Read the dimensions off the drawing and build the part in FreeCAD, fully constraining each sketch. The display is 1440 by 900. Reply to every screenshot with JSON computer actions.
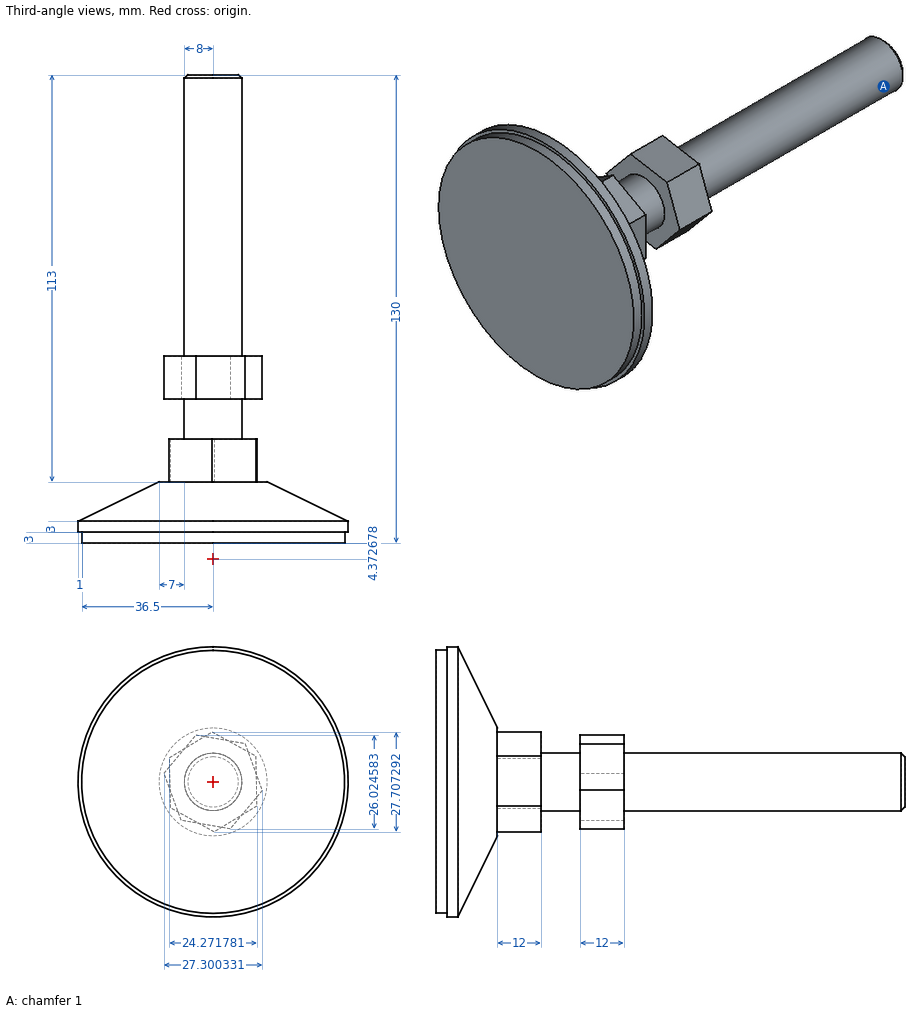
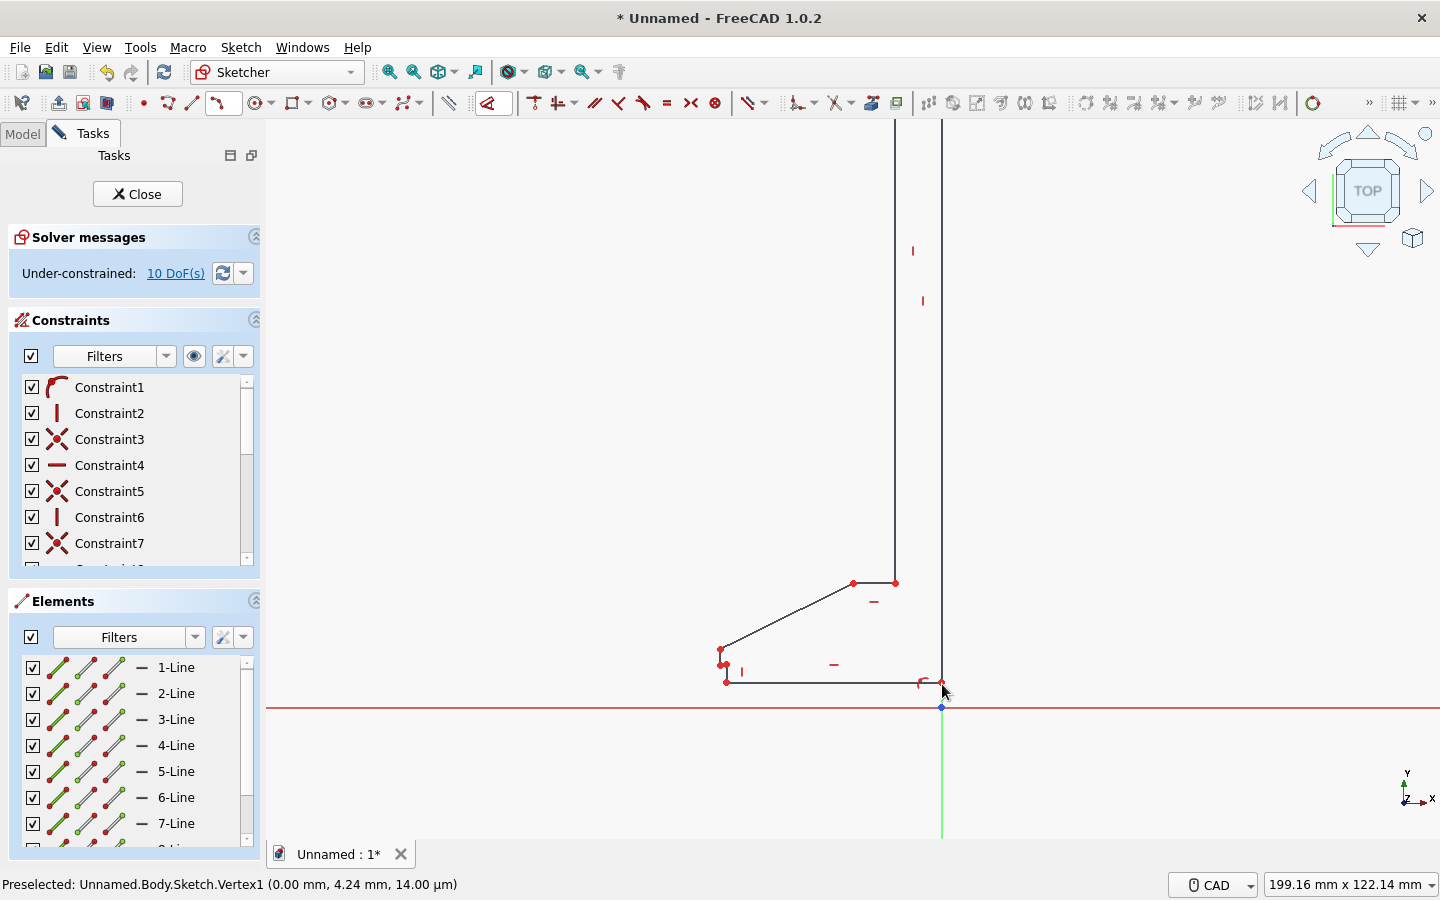
{"action": "scroll", "coordinate": [723, 665], "scroll_direction": "up", "scroll_amount": 8}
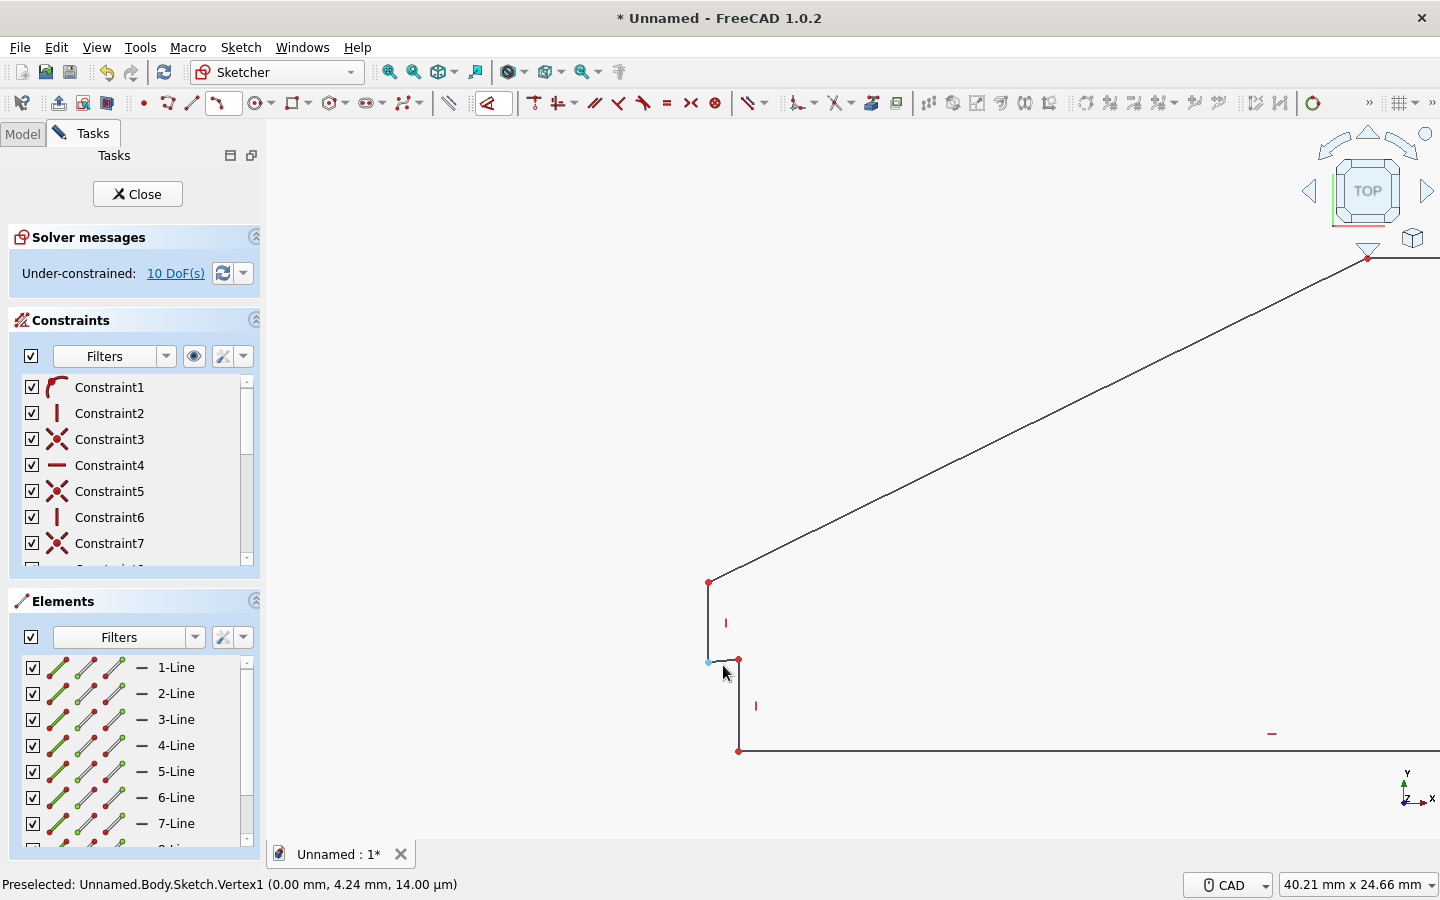
{"action": "left_click", "coordinate": [724, 661]}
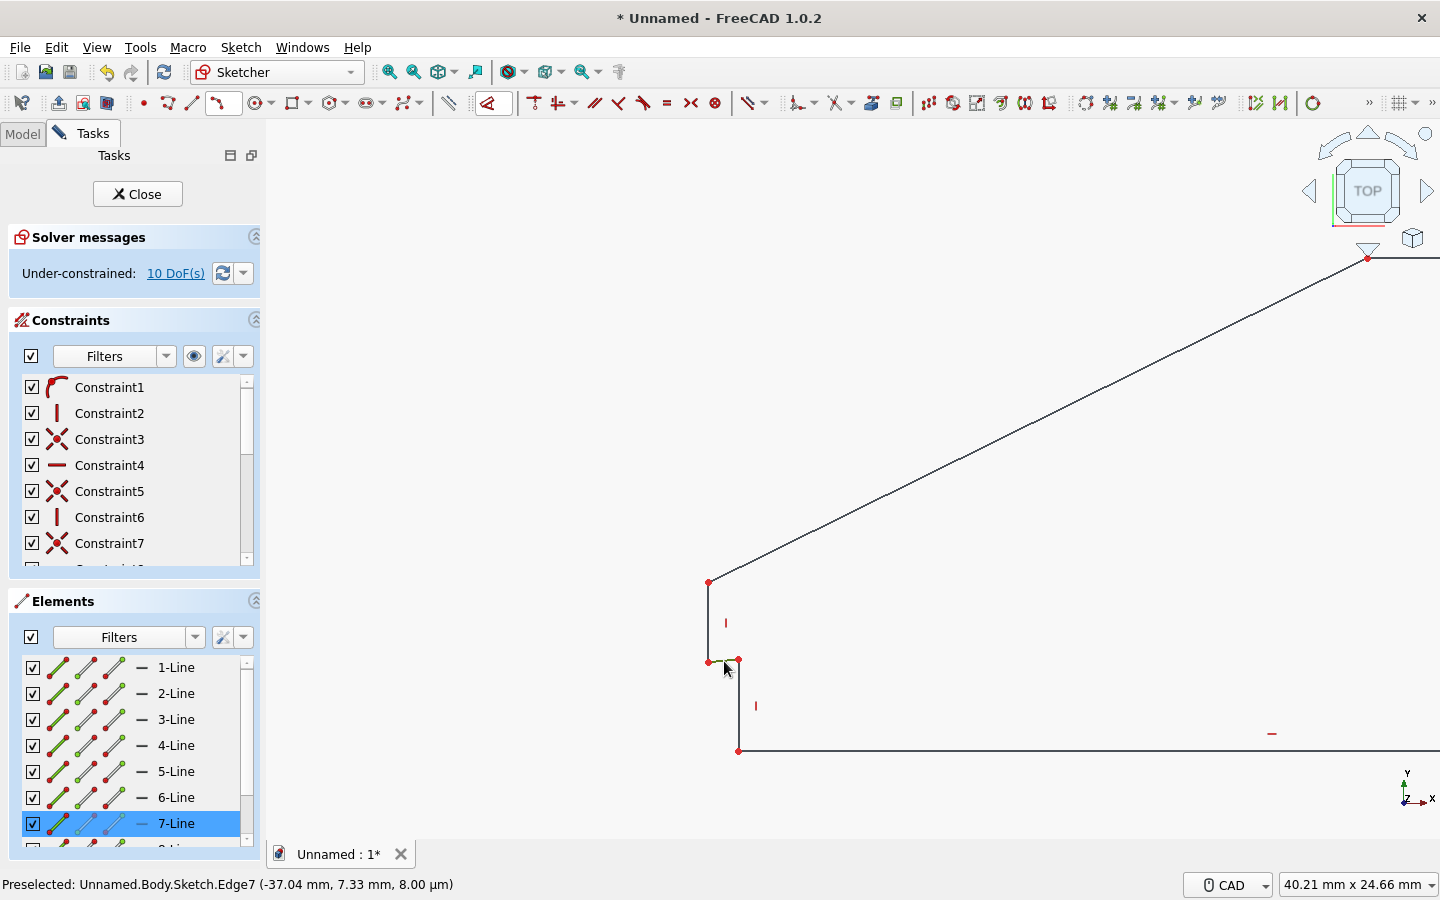
{"action": "key", "text": "h"}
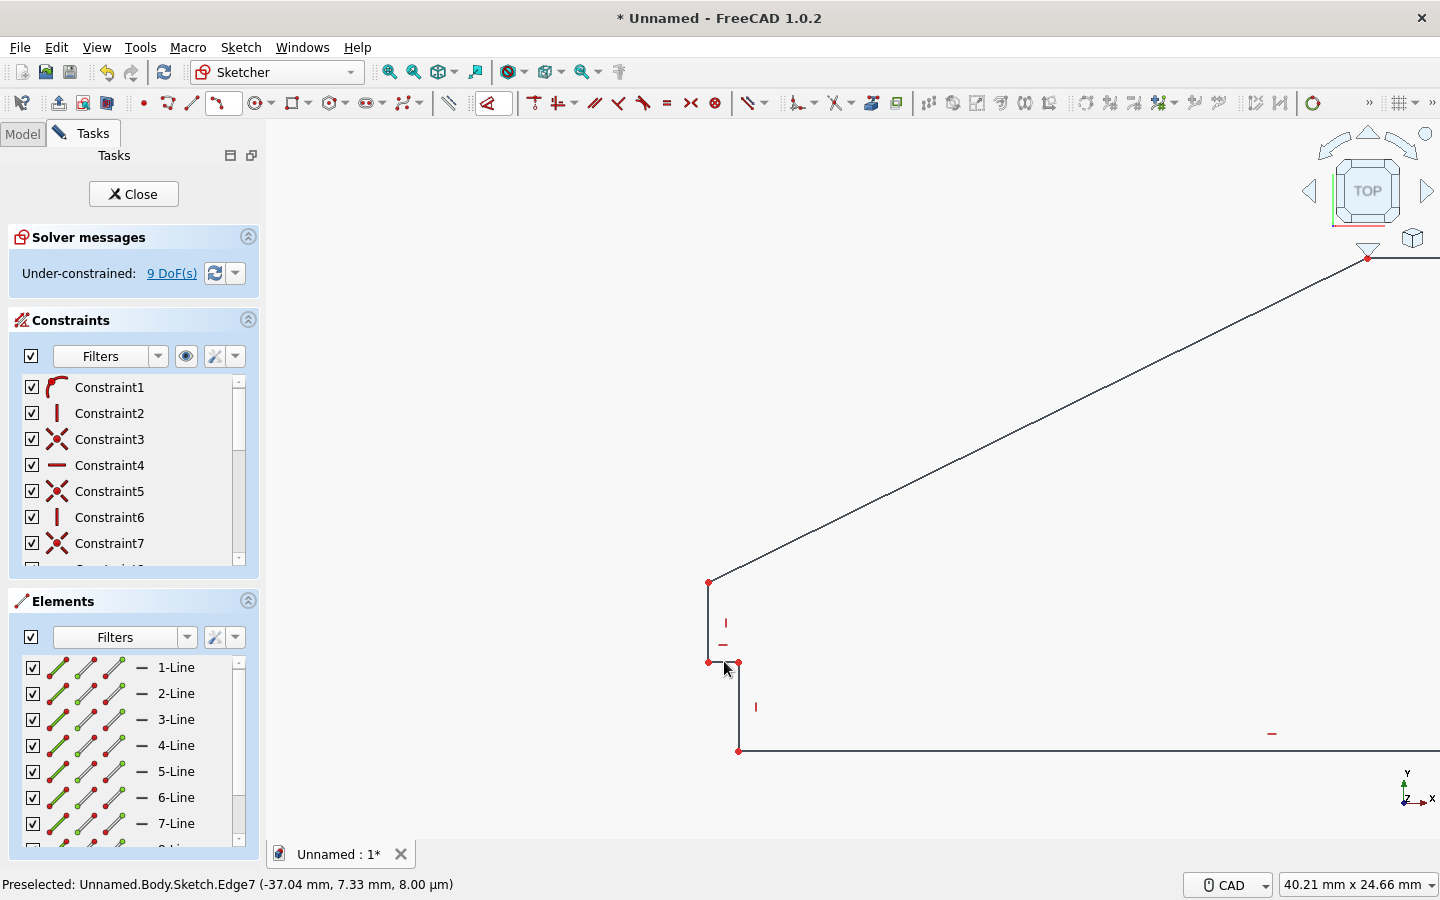
{"action": "scroll", "coordinate": [726, 674], "scroll_direction": "down", "scroll_amount": 11}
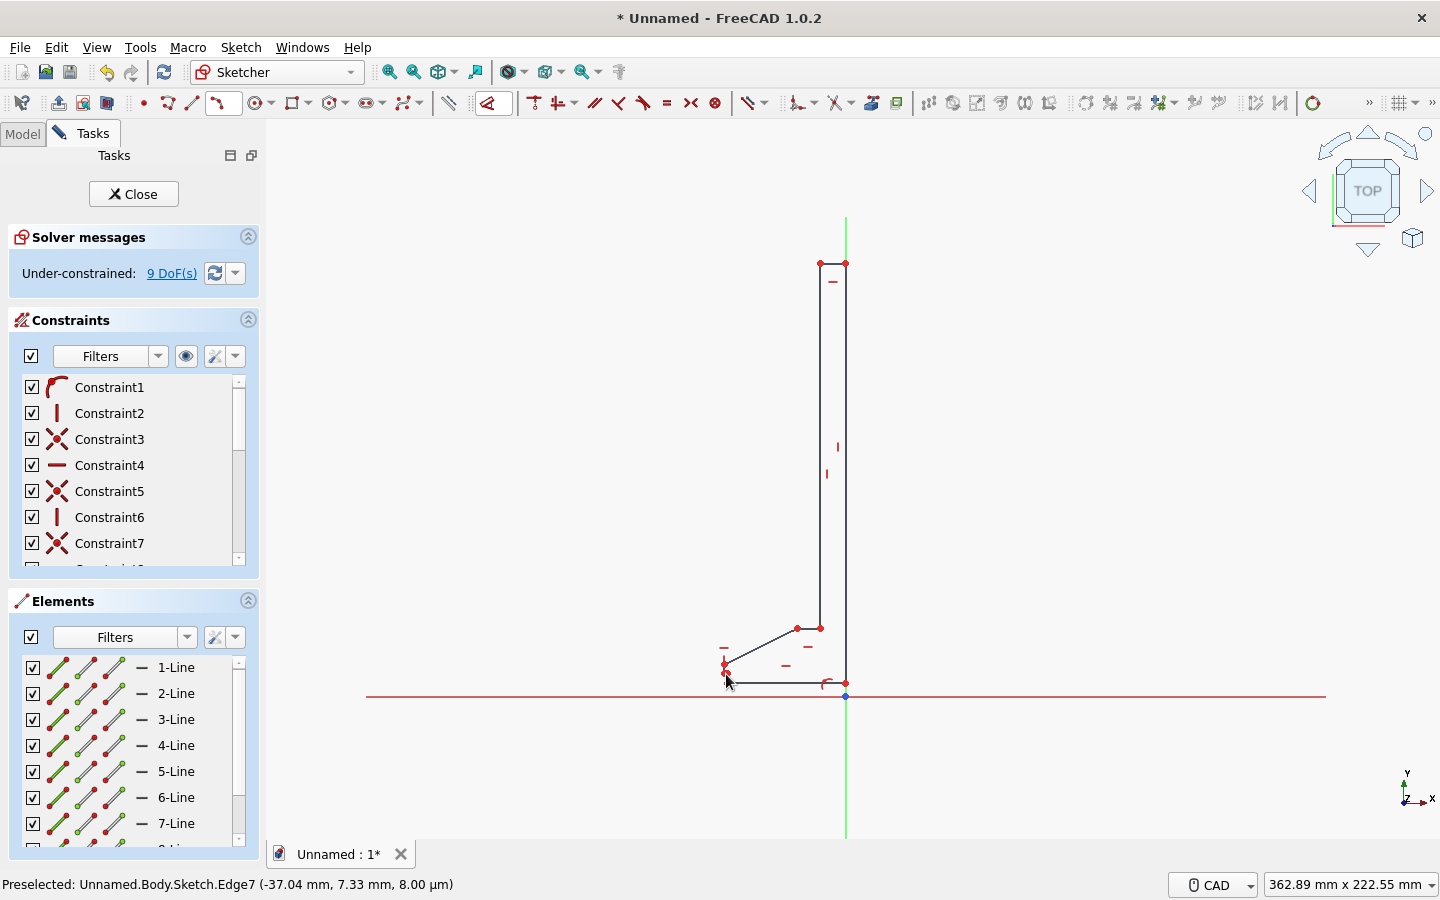
{"action": "scroll", "coordinate": [838, 264], "scroll_direction": "up", "scroll_amount": 3}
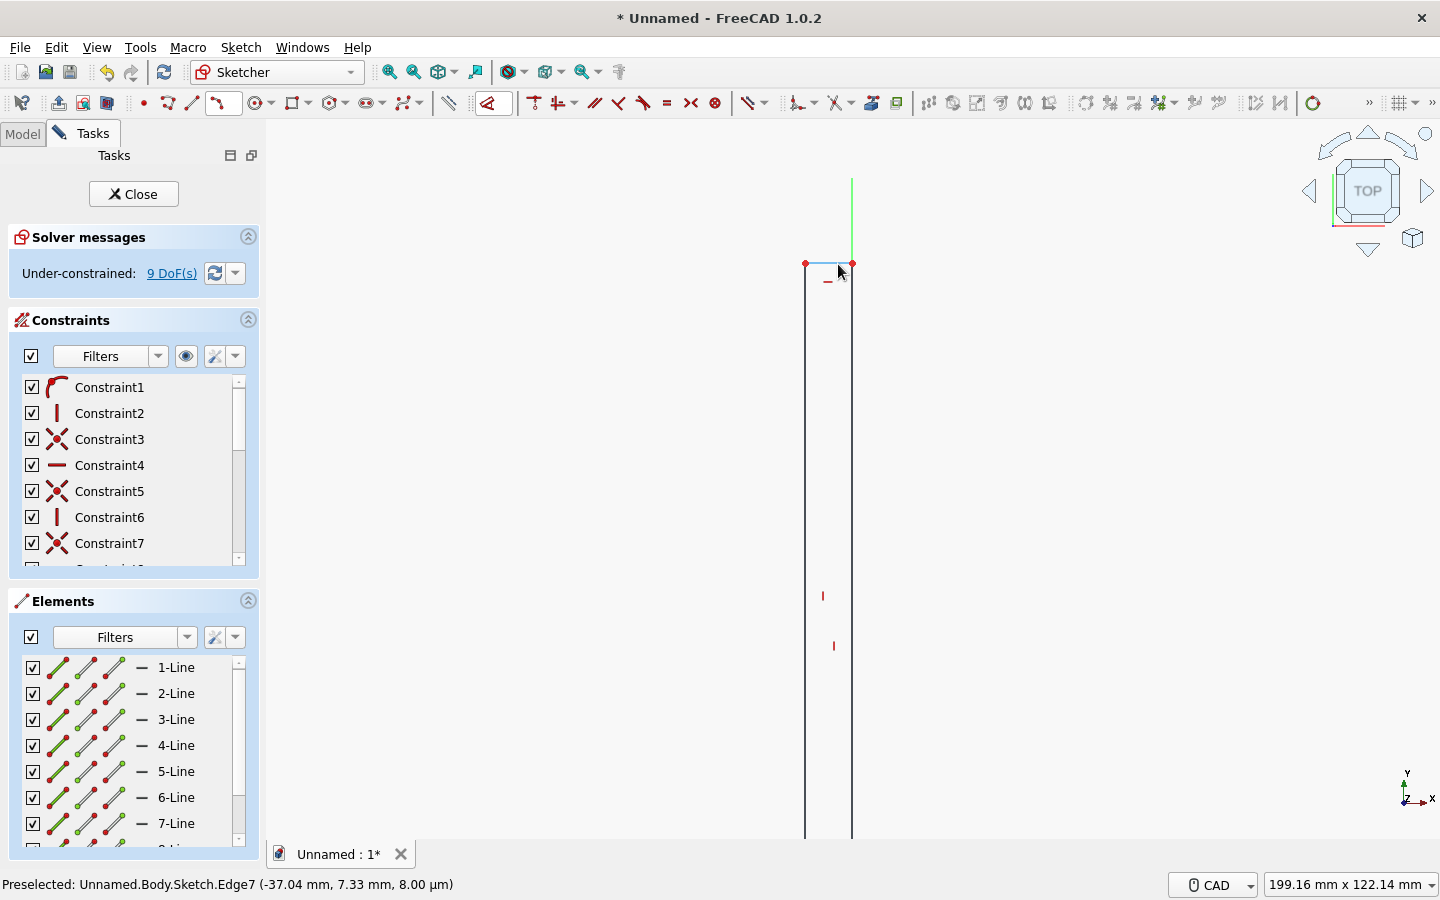
{"action": "left_click", "coordinate": [838, 263]}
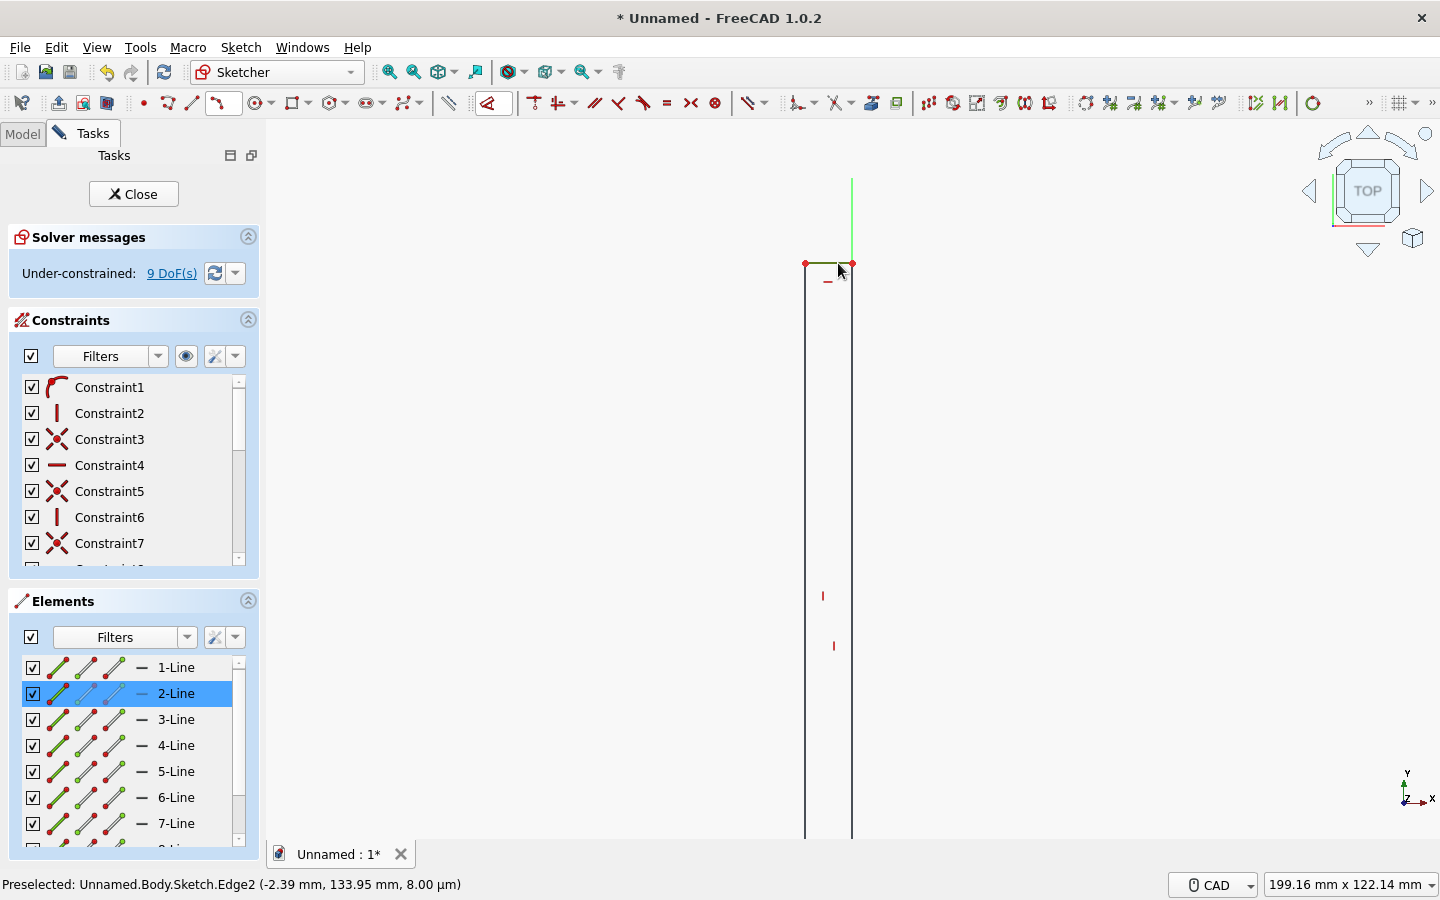
{"action": "left_click", "coordinate": [506, 104]}